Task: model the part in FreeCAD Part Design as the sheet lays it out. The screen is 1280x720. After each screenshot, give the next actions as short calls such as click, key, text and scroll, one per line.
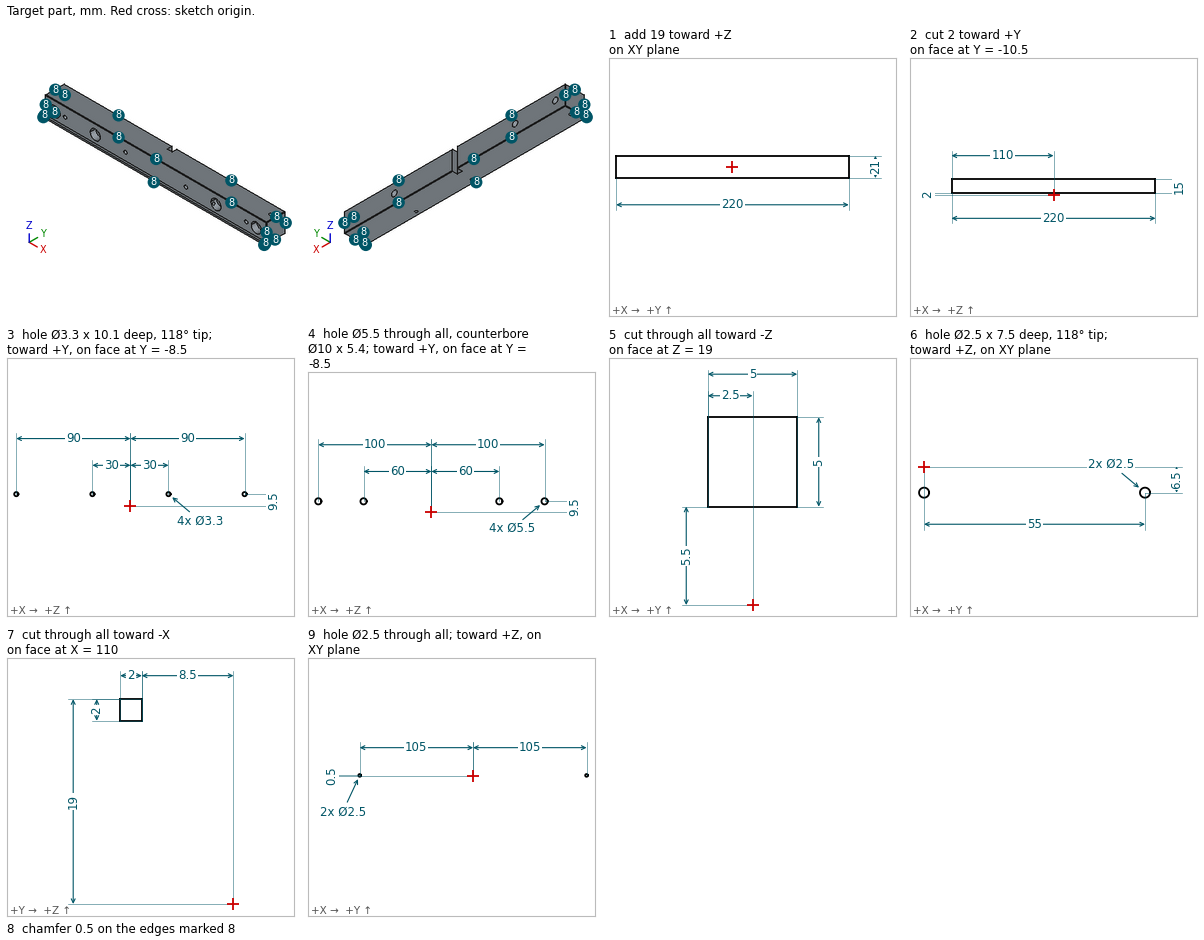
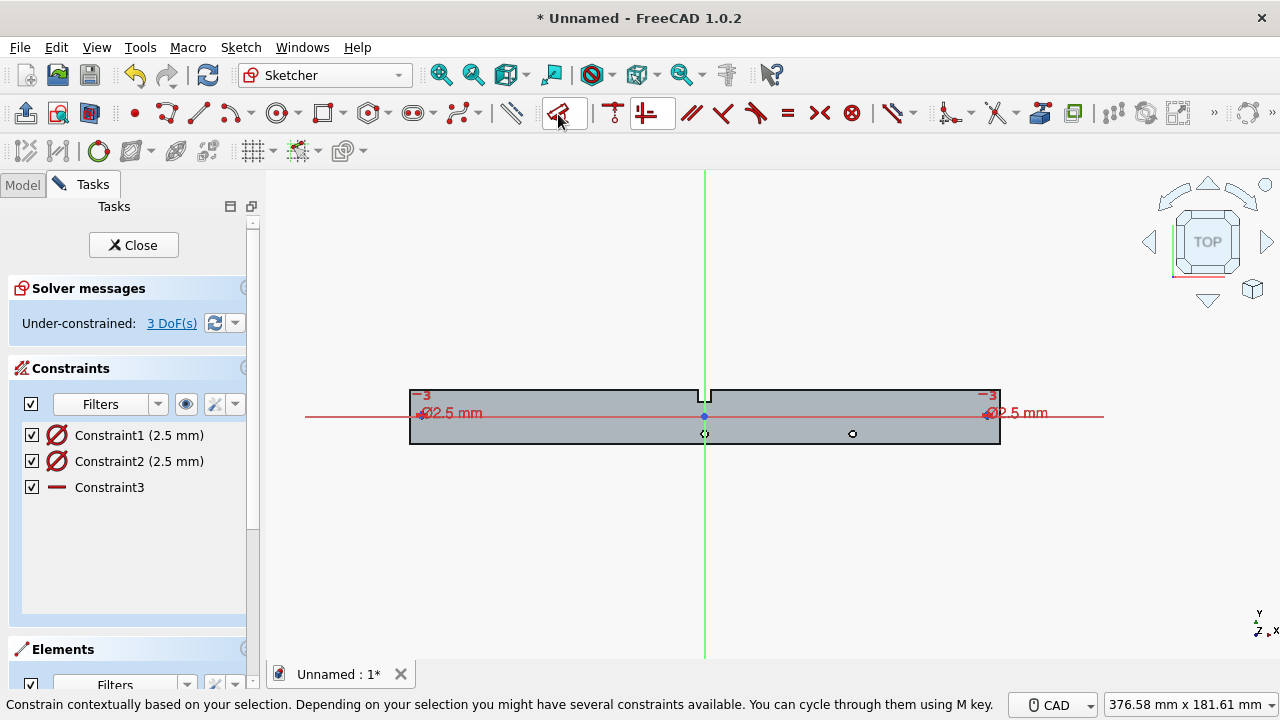
click(422, 415)
click(563, 451)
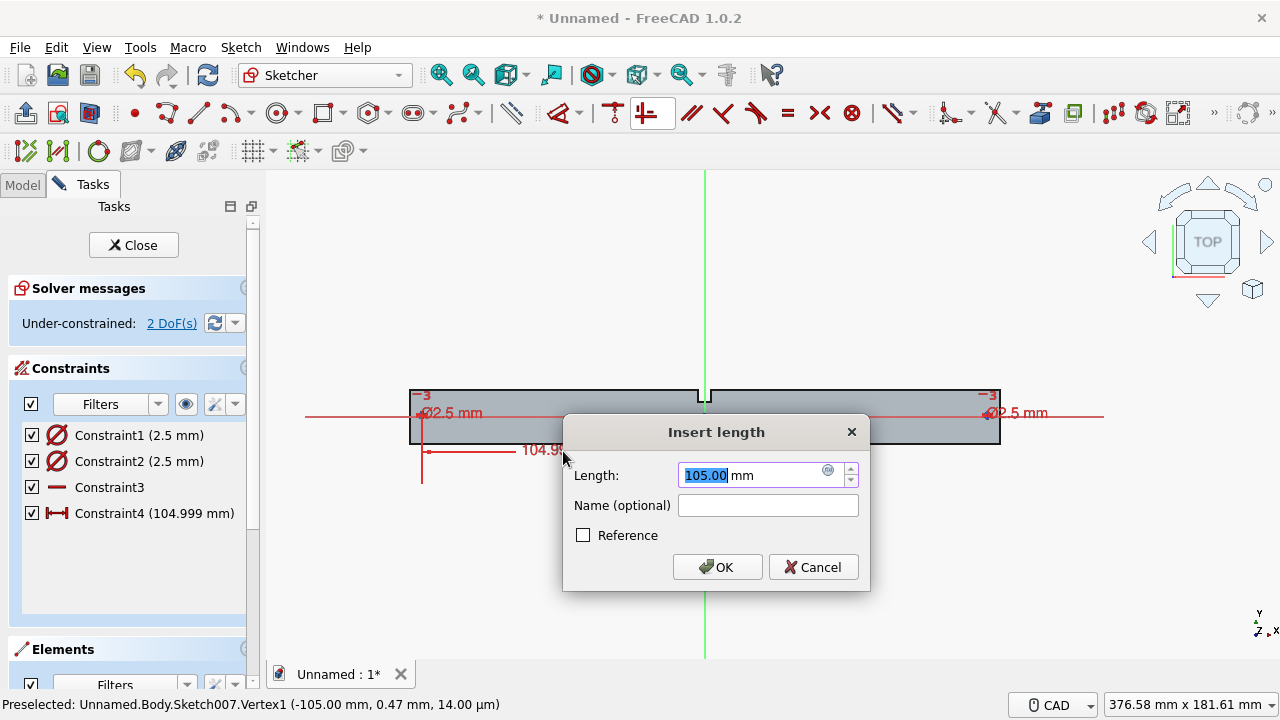
text(105)
key(Return)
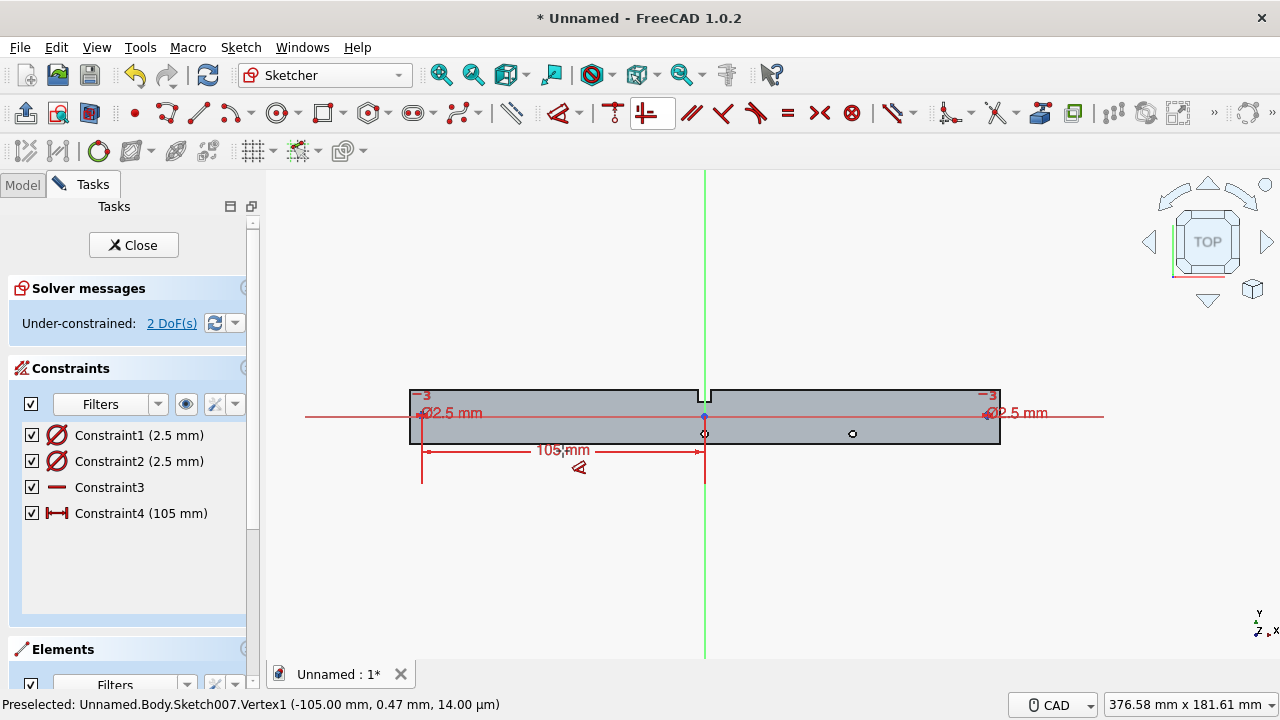
scroll(422, 415, up, 17)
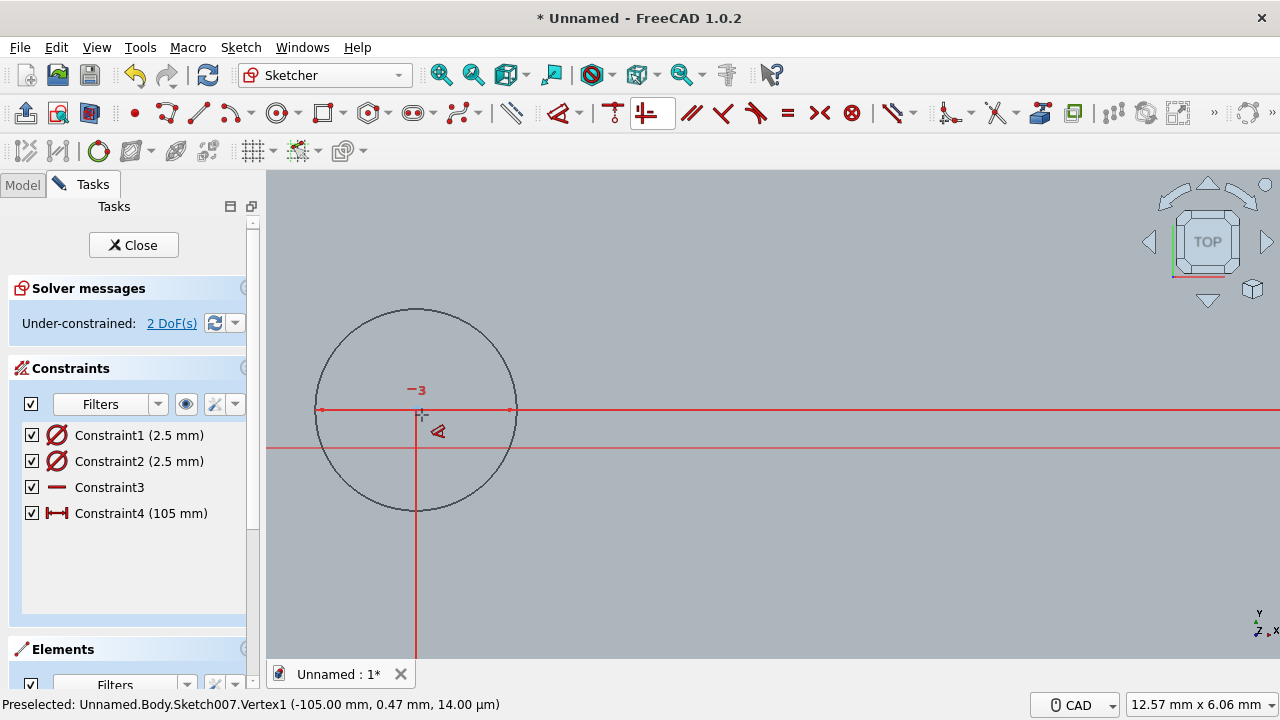
click(416, 410)
click(382, 429)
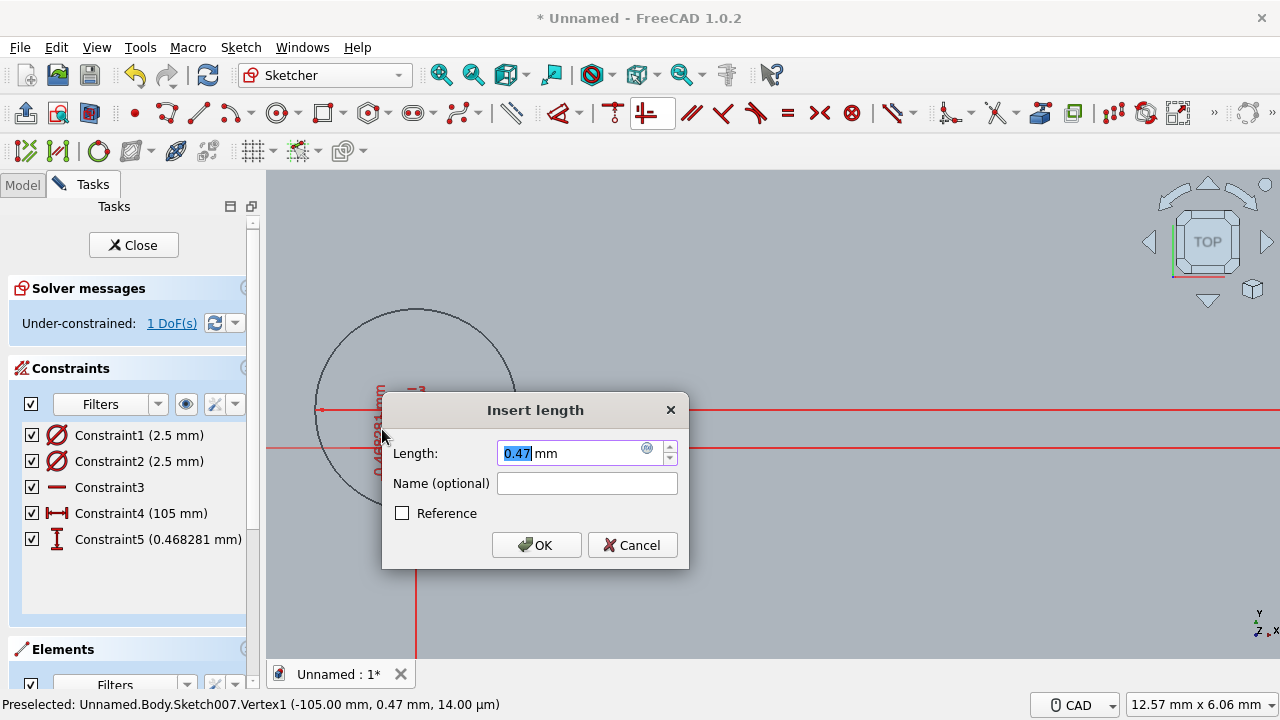
text(0.5)
key(Return)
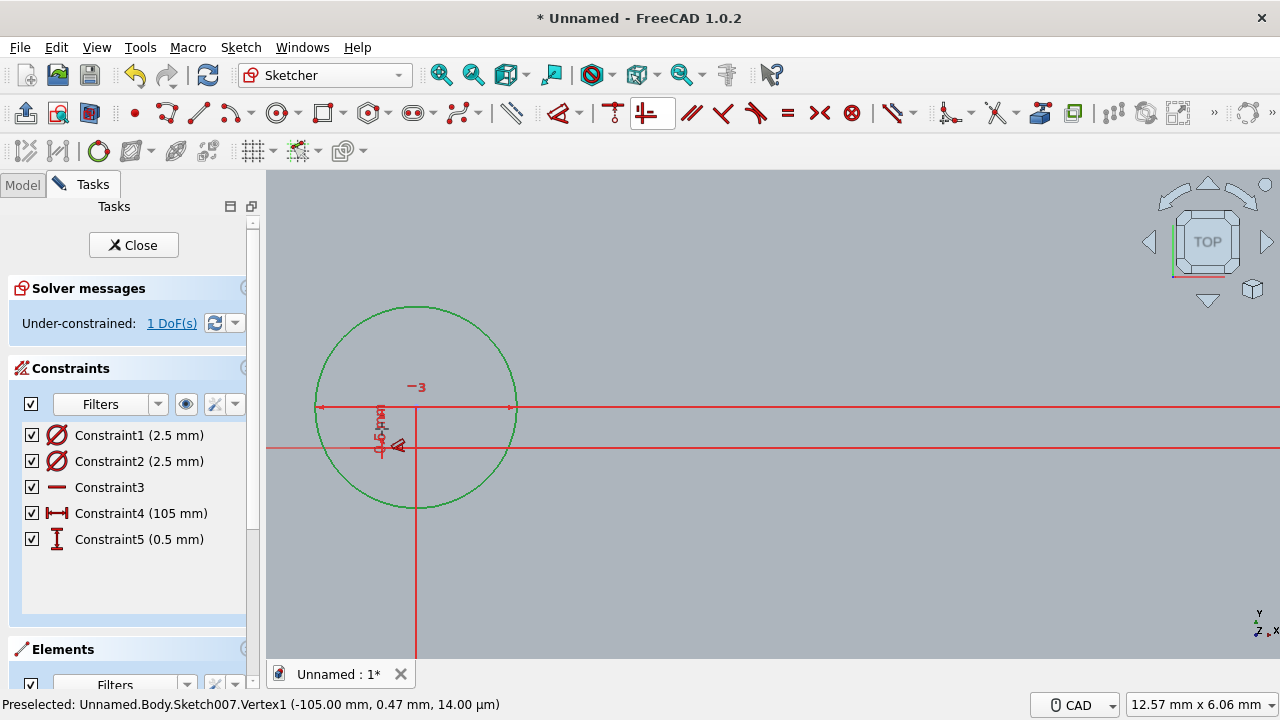
scroll(357, 415, down, 16)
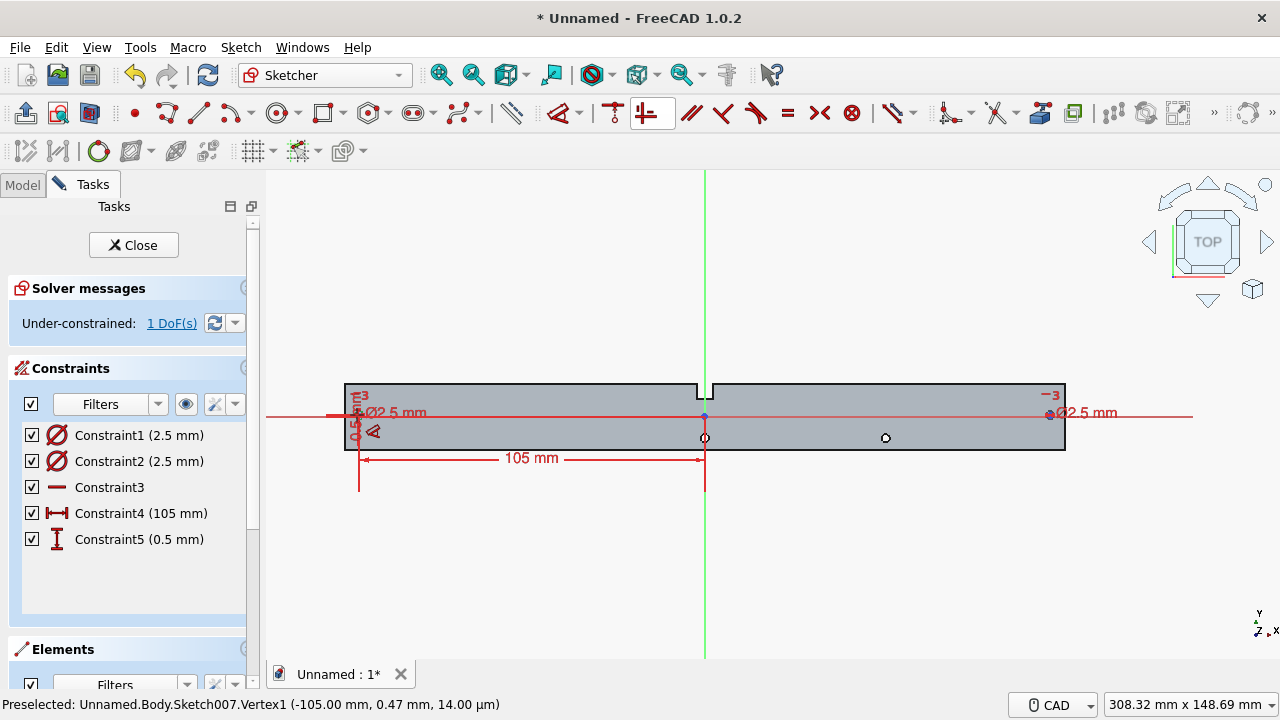
click(1050, 415)
click(877, 451)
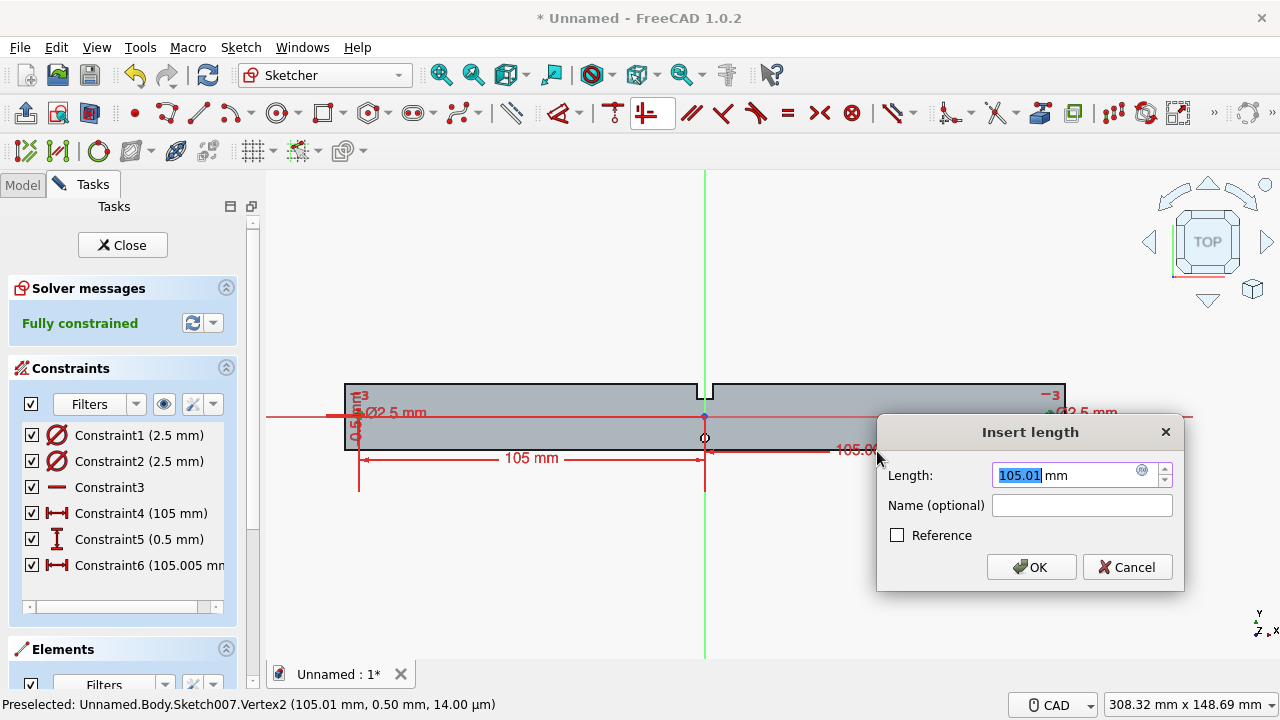
text(105)
key(Return)
key(Escape)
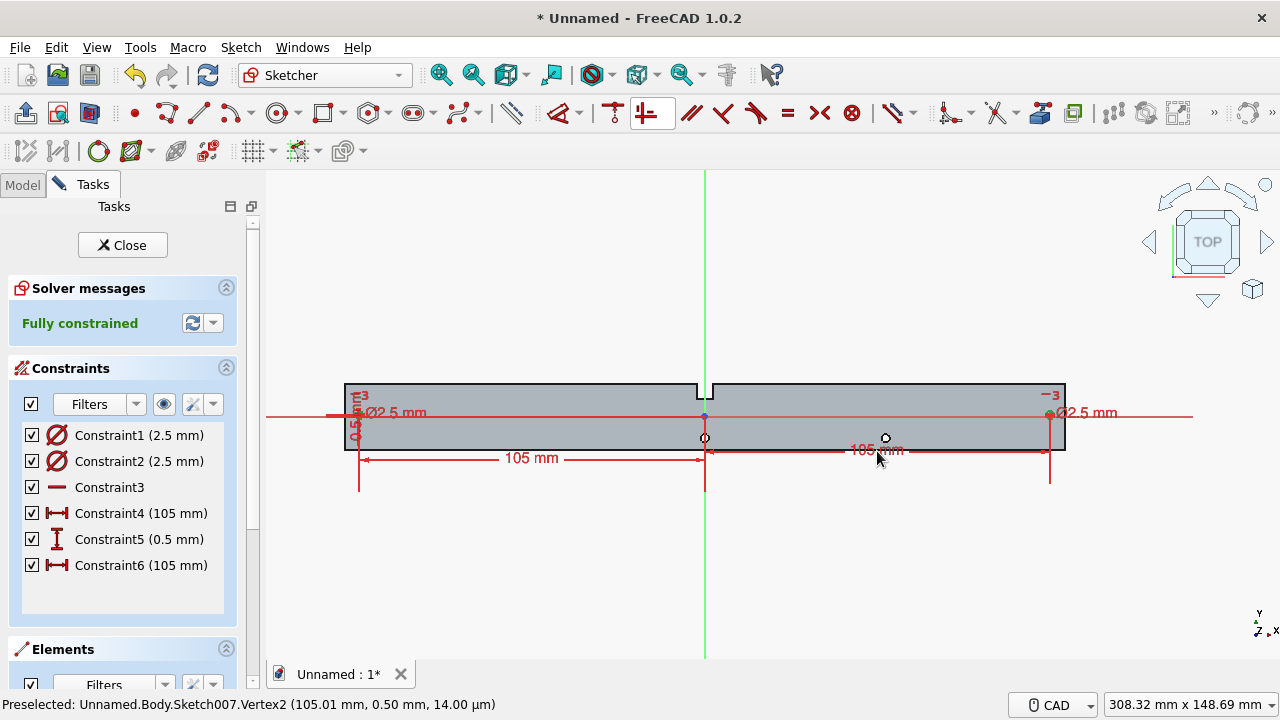
click(123, 245)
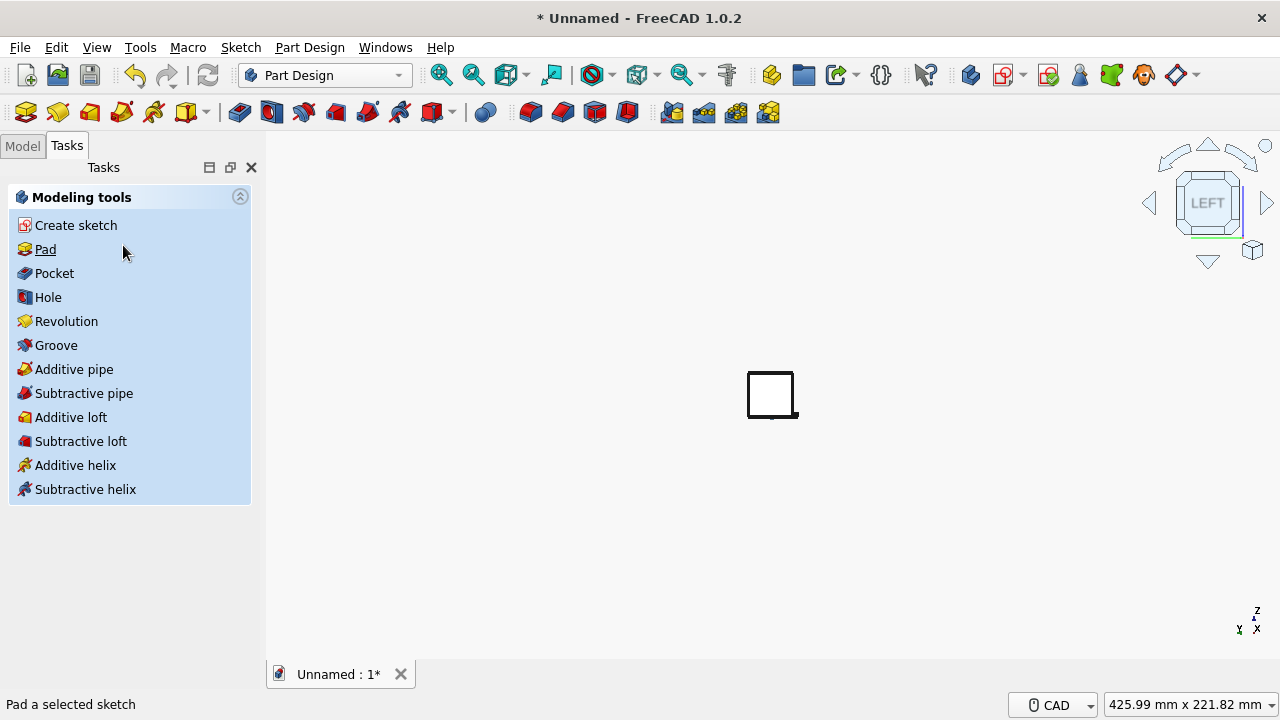
click(272, 112)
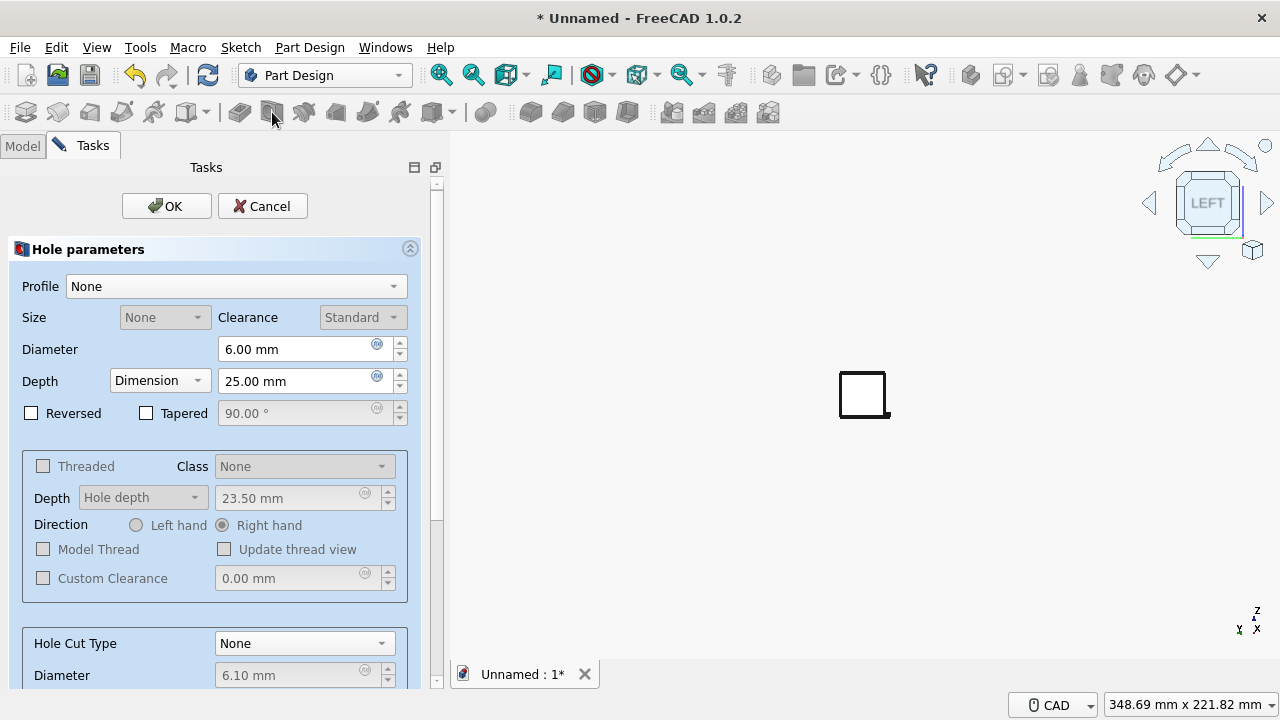
triple_click(305, 349)